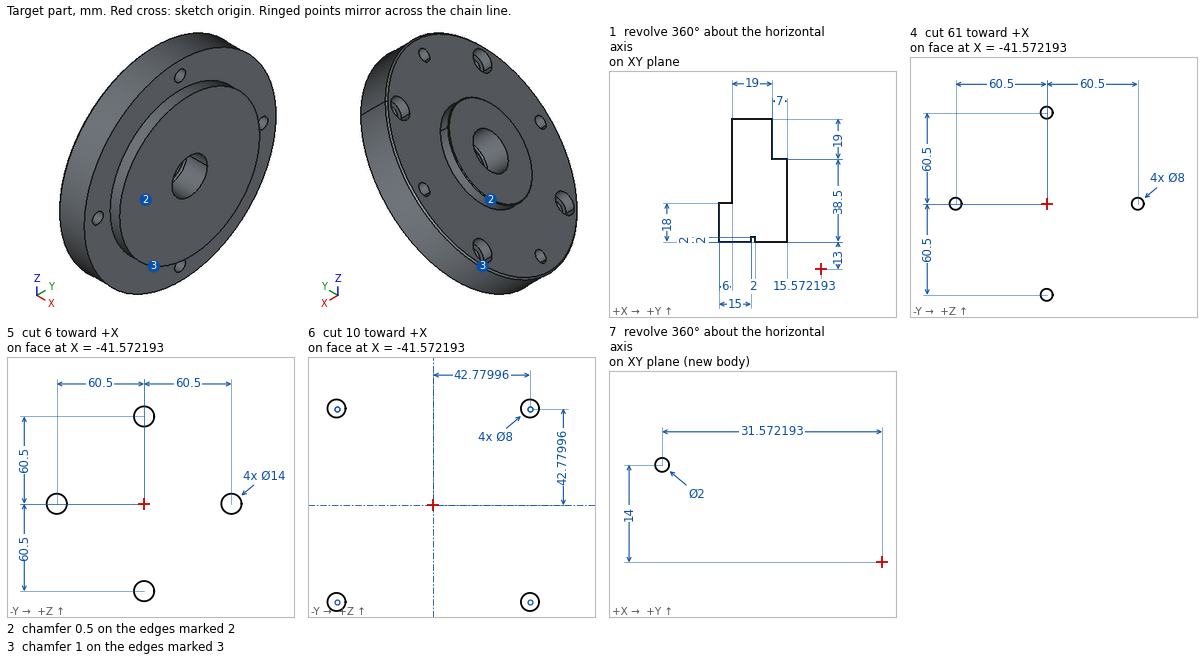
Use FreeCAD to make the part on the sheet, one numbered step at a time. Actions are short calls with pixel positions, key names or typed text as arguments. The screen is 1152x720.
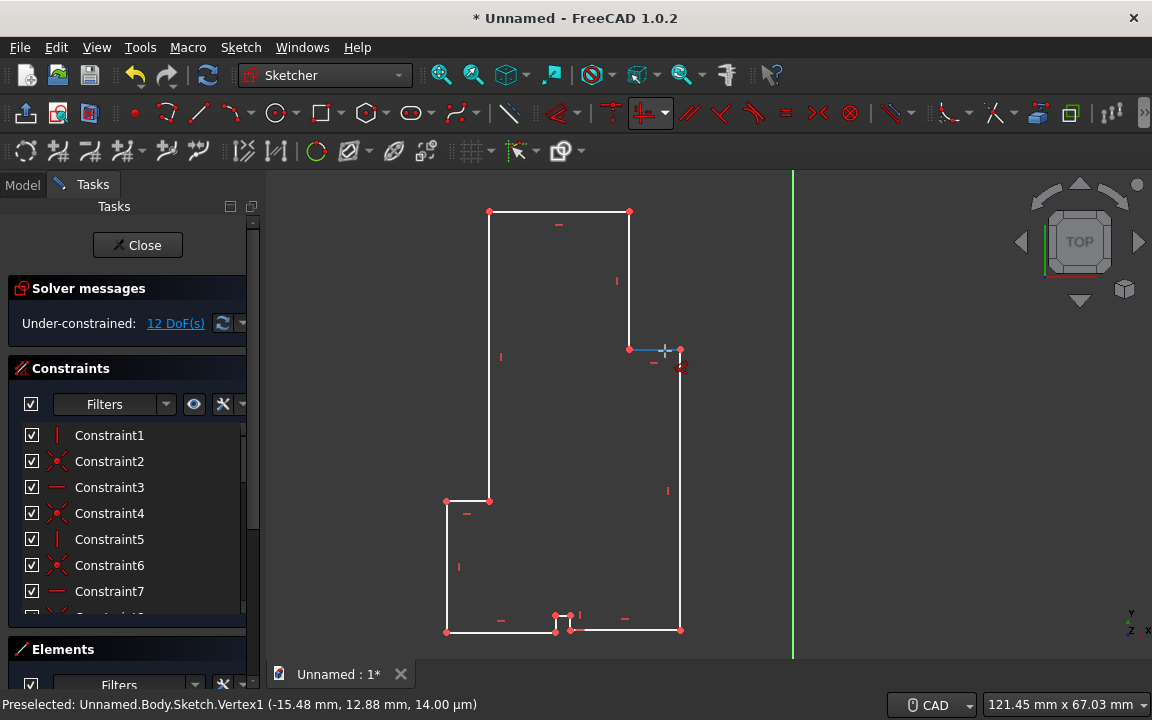
click(665, 350)
click(655, 316)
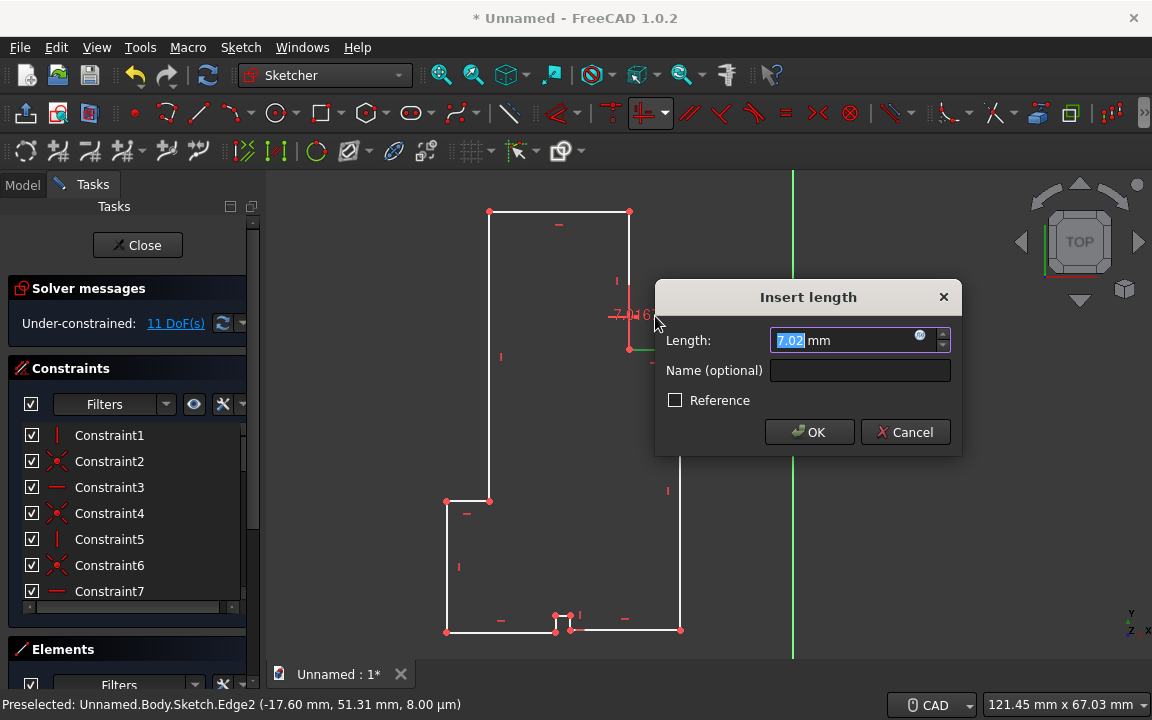
text(7)
key(Return)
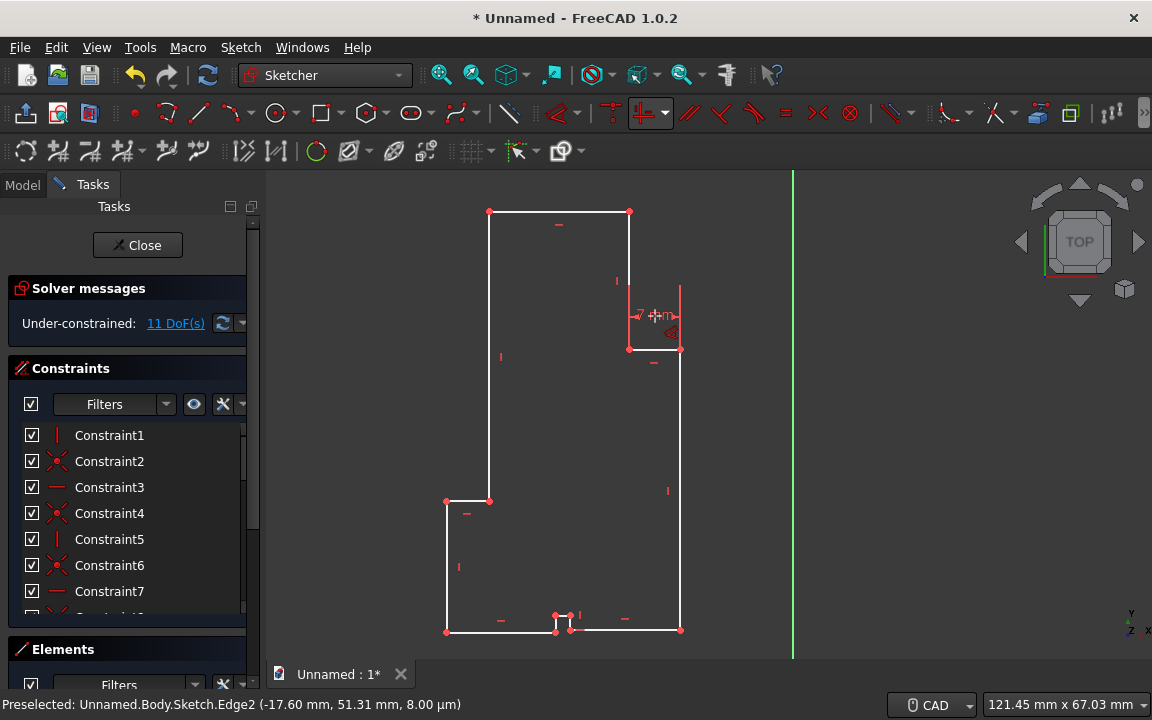
click(476, 501)
click(468, 535)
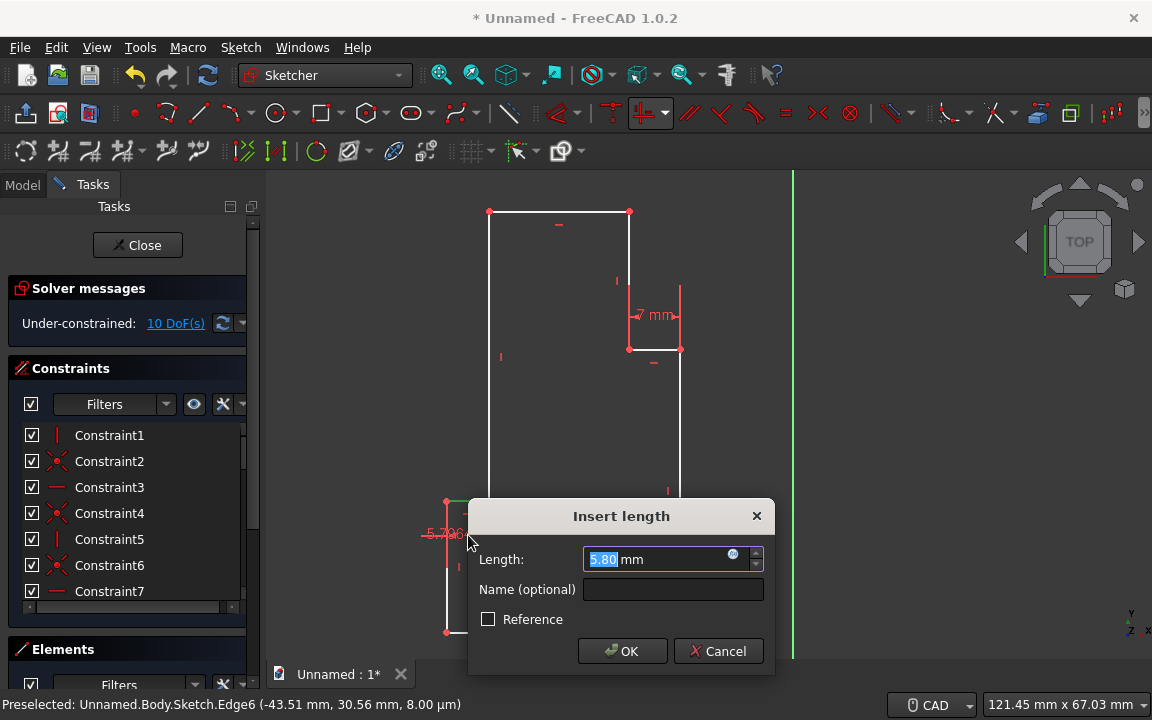
text(6)
key(Return)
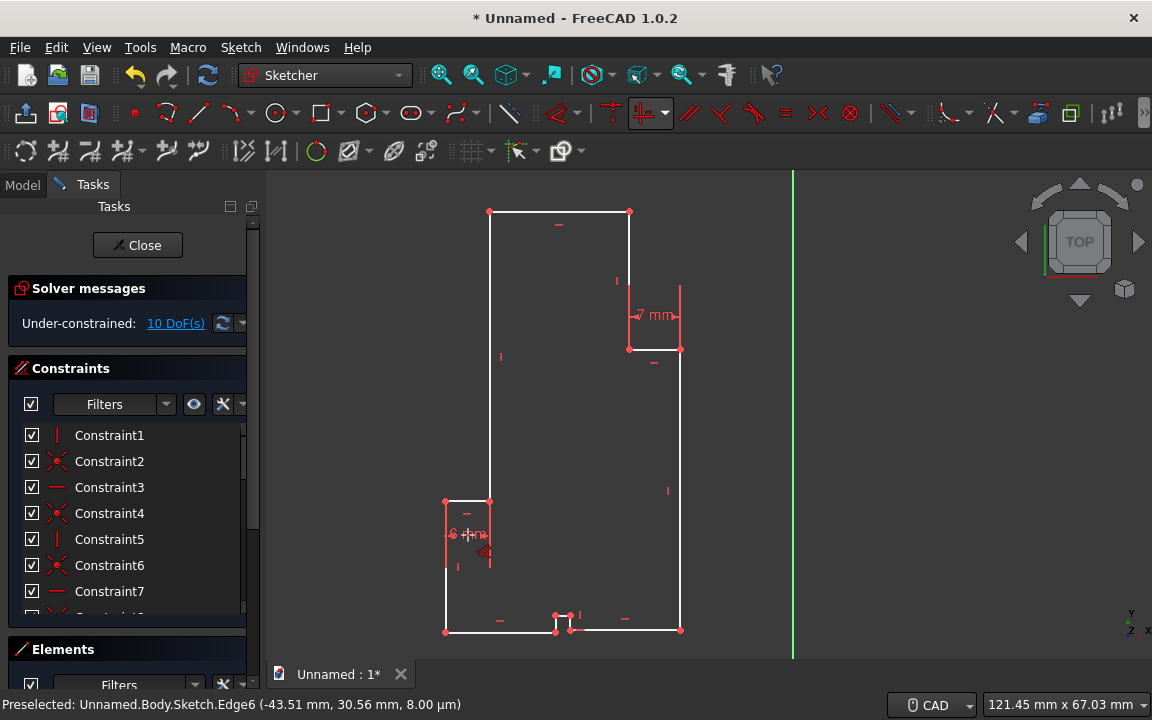
scroll(556, 624, up, 6)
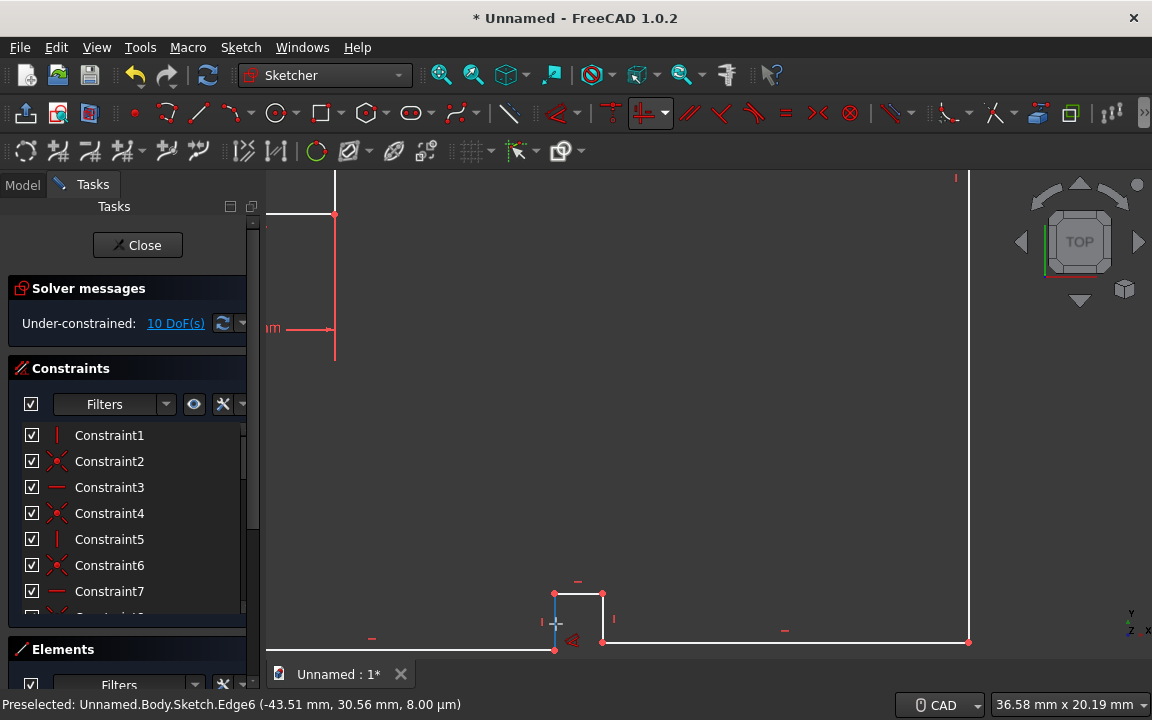
click(555, 622)
click(521, 612)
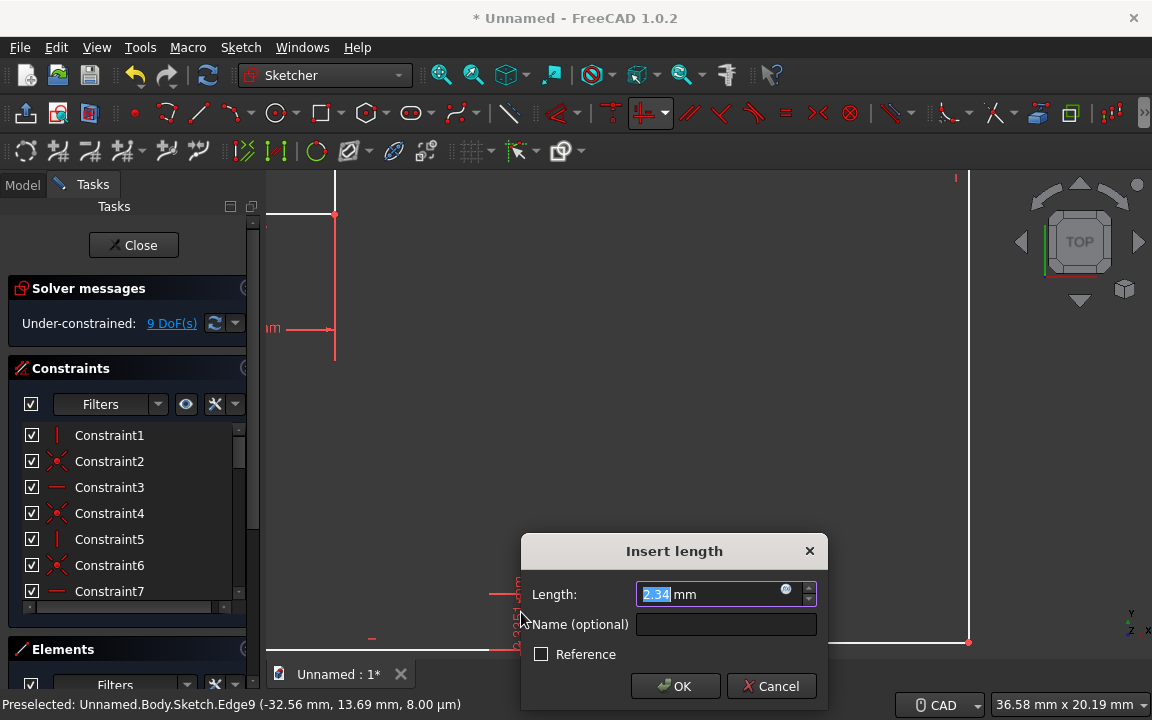
text(2)
key(Return)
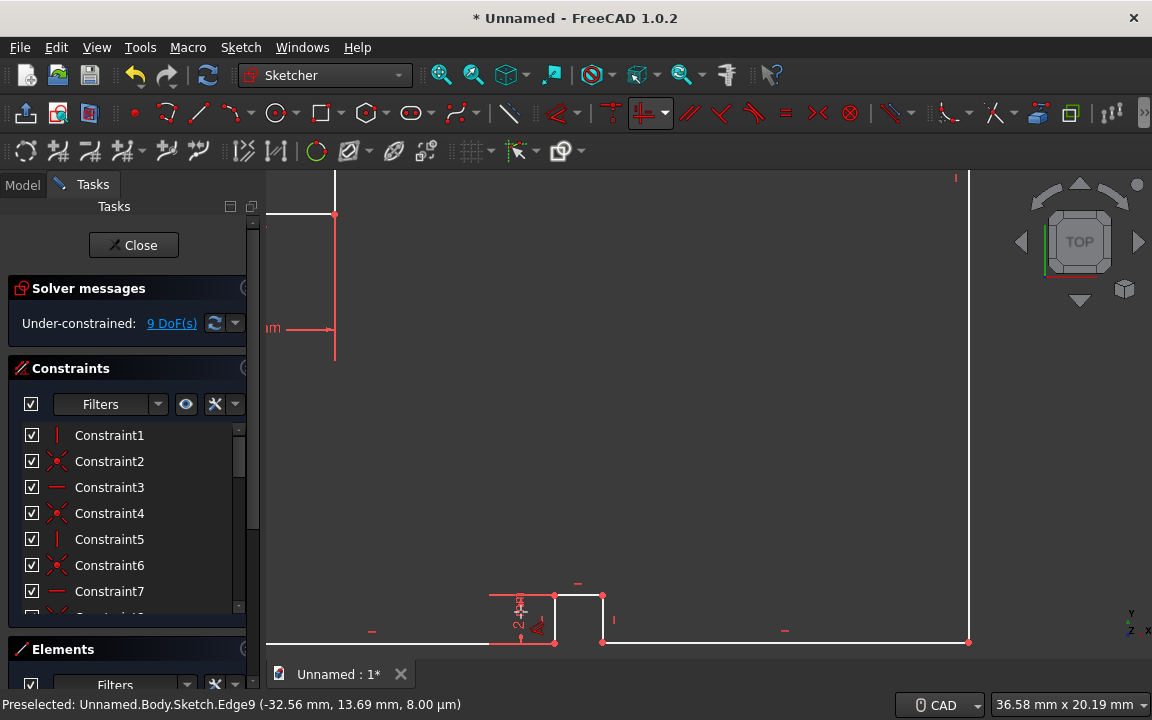
click(569, 595)
click(579, 561)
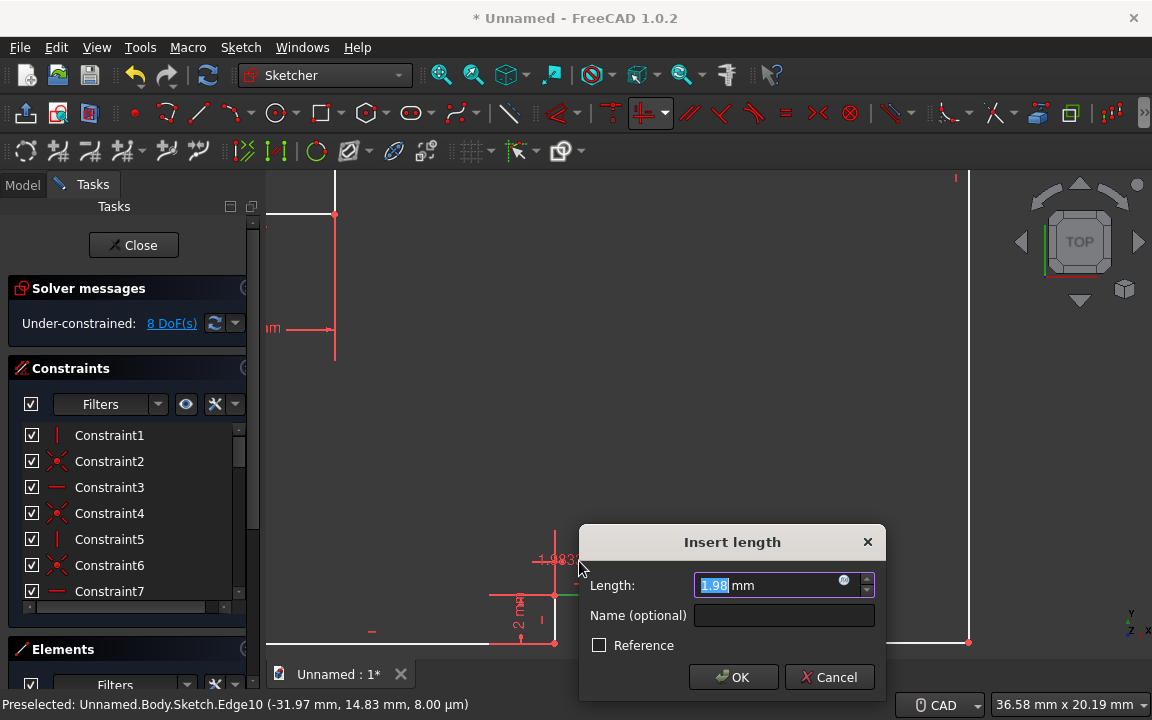
text(2)
key(Return)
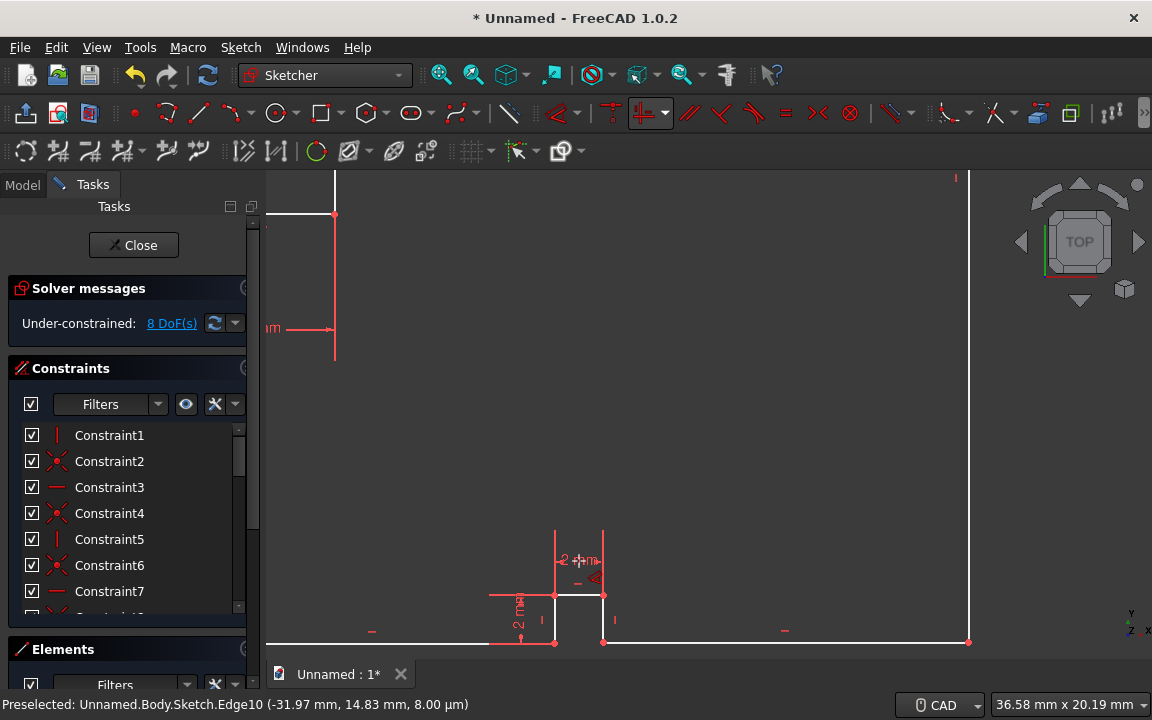
click(603, 610)
click(637, 613)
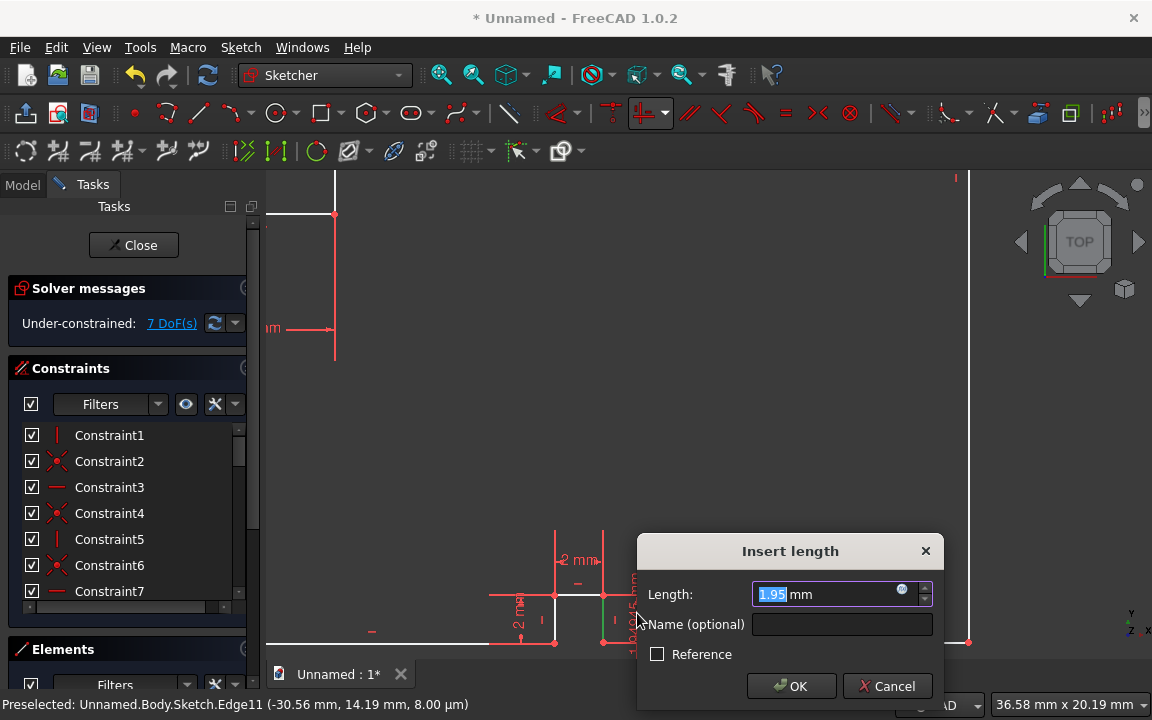
text(2)
key(Return)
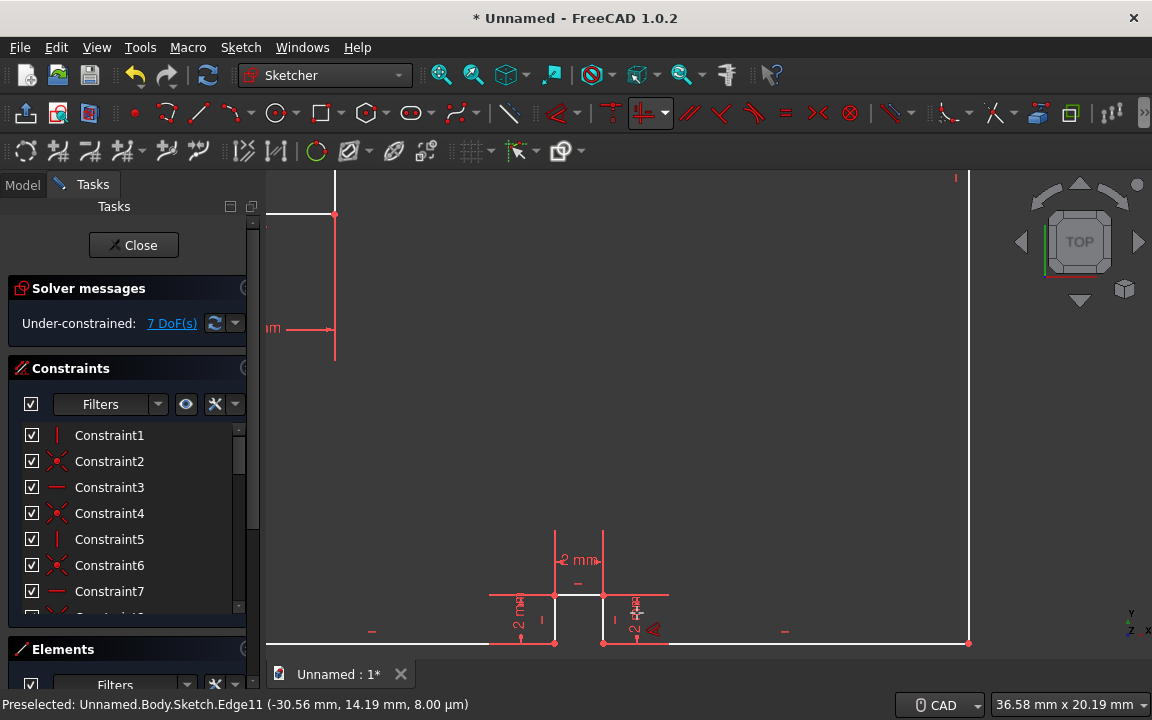
scroll(615, 477, down, 9)